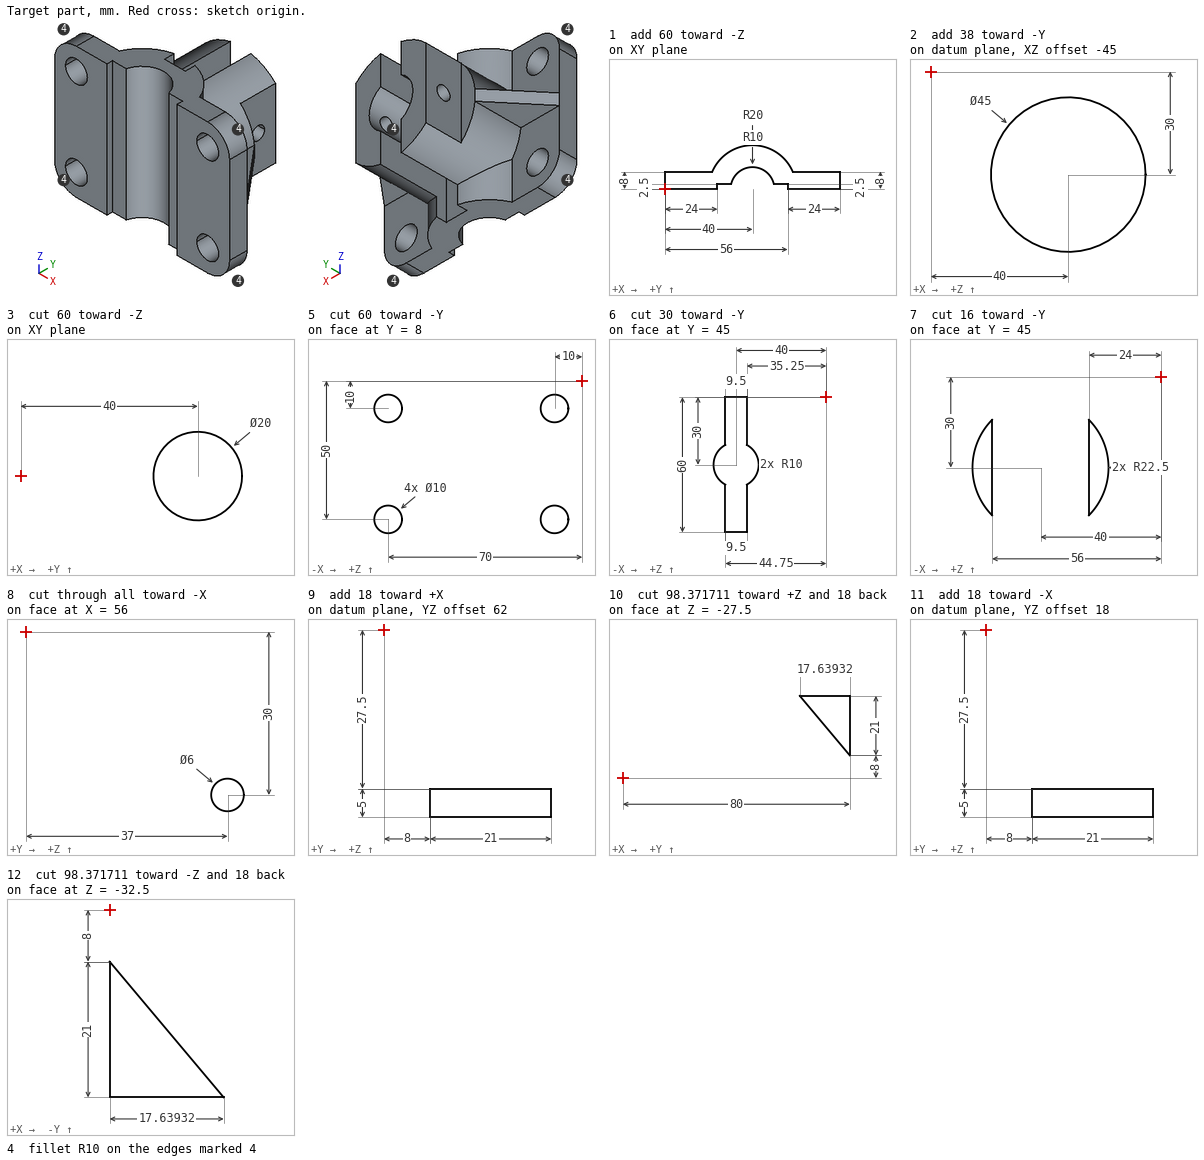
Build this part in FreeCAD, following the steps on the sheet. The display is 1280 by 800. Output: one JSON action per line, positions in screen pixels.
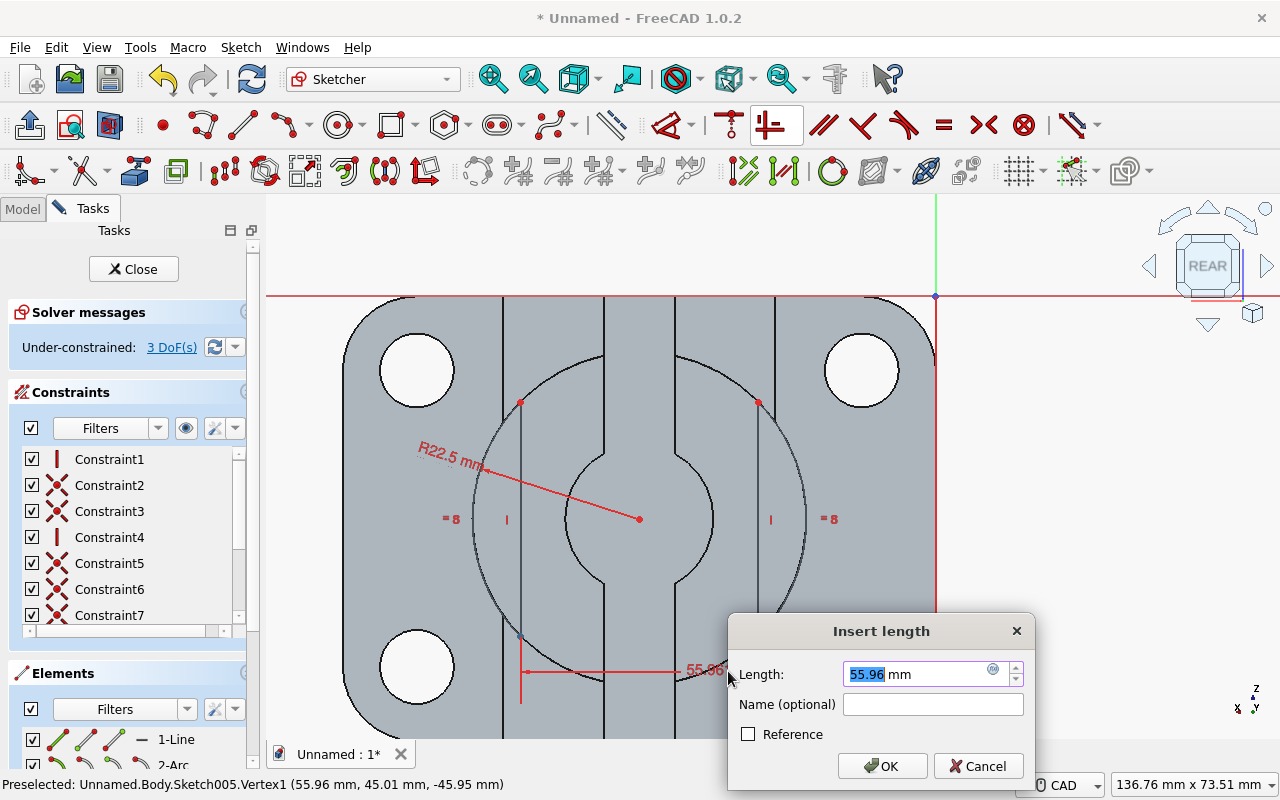
{"action": "type", "text": "56"}
{"action": "key", "text": "Return"}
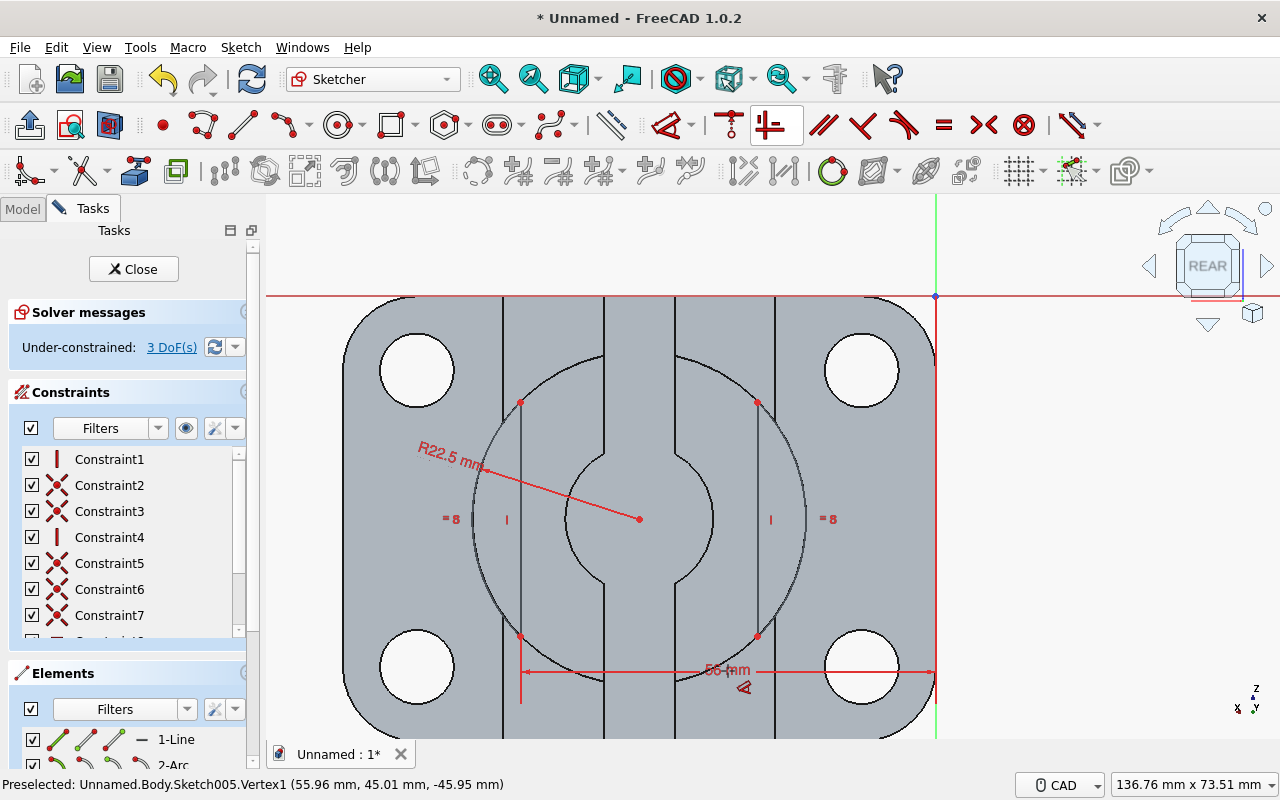
{"action": "left_click", "coordinate": [758, 402]}
{"action": "left_click", "coordinate": [847, 262]}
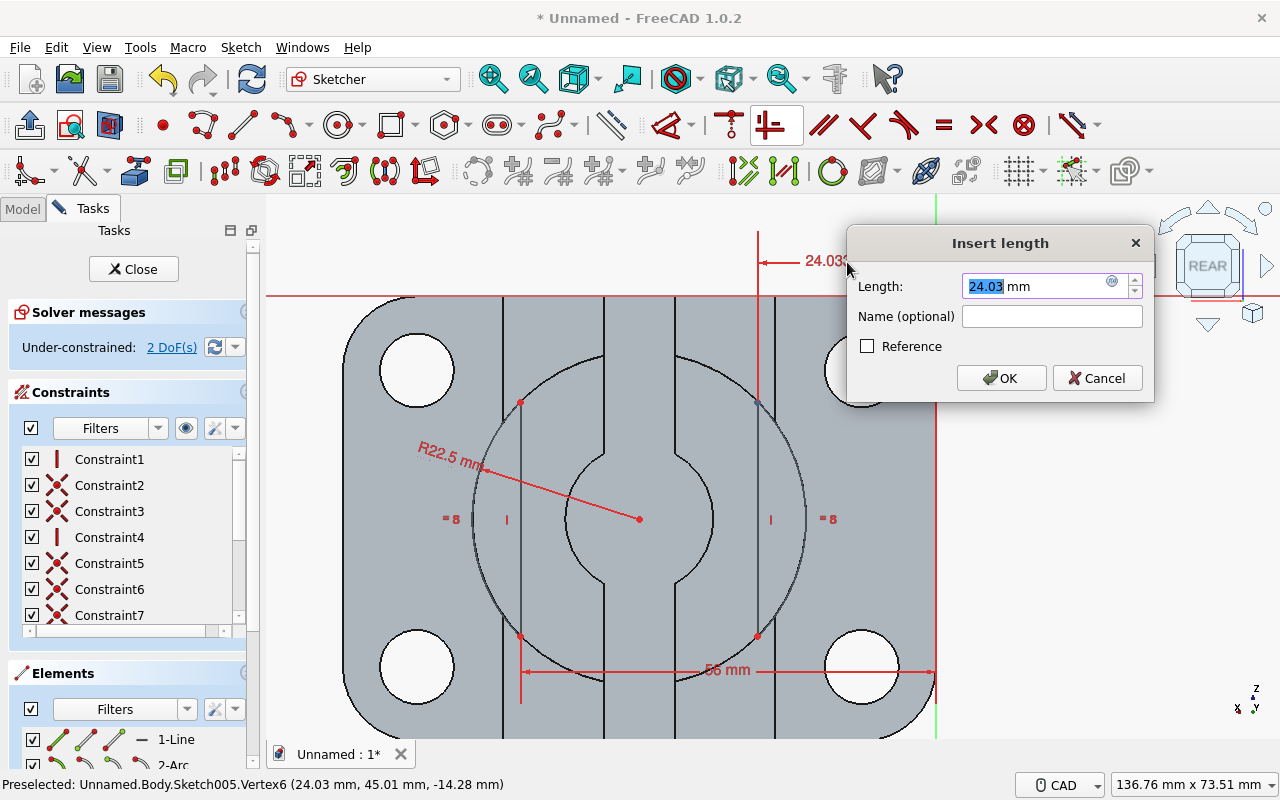
{"action": "type", "text": "24"}
{"action": "key", "text": "Return"}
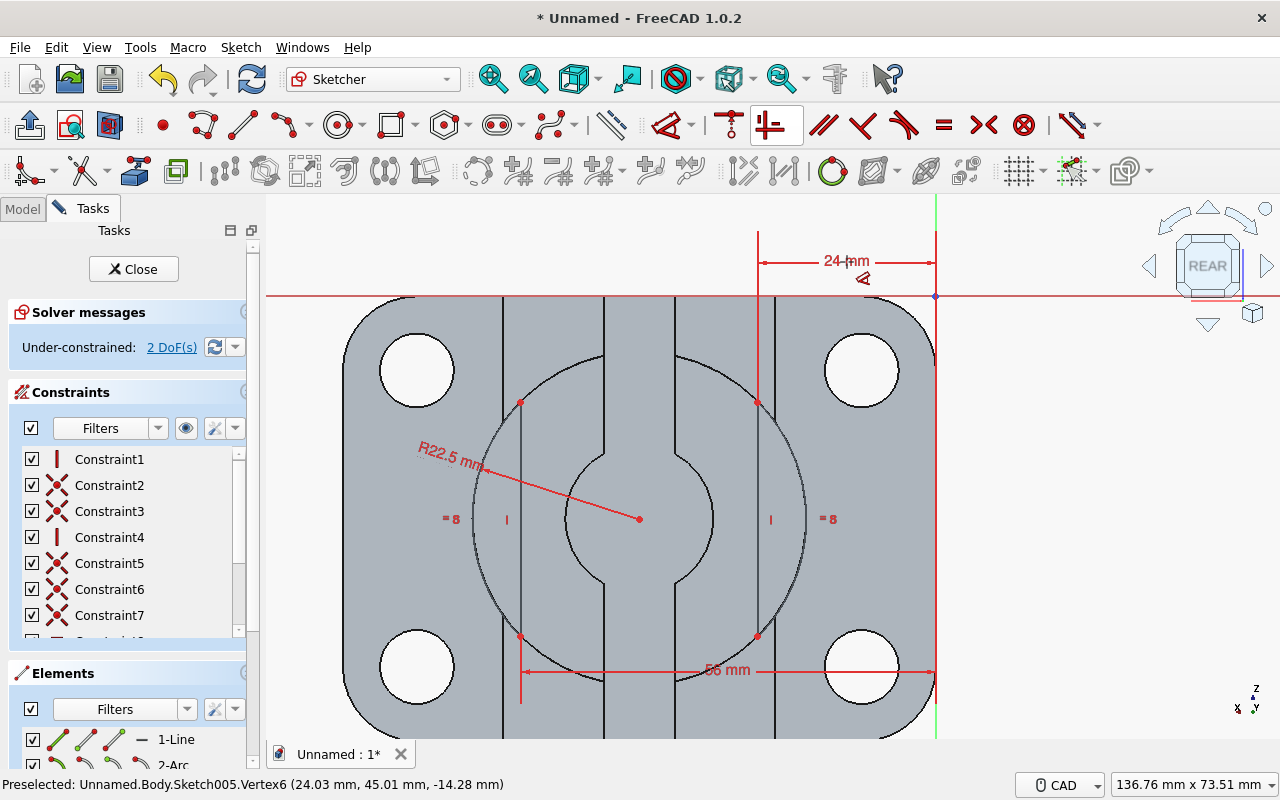
{"action": "left_click", "coordinate": [639, 520]}
{"action": "left_click", "coordinate": [719, 262]}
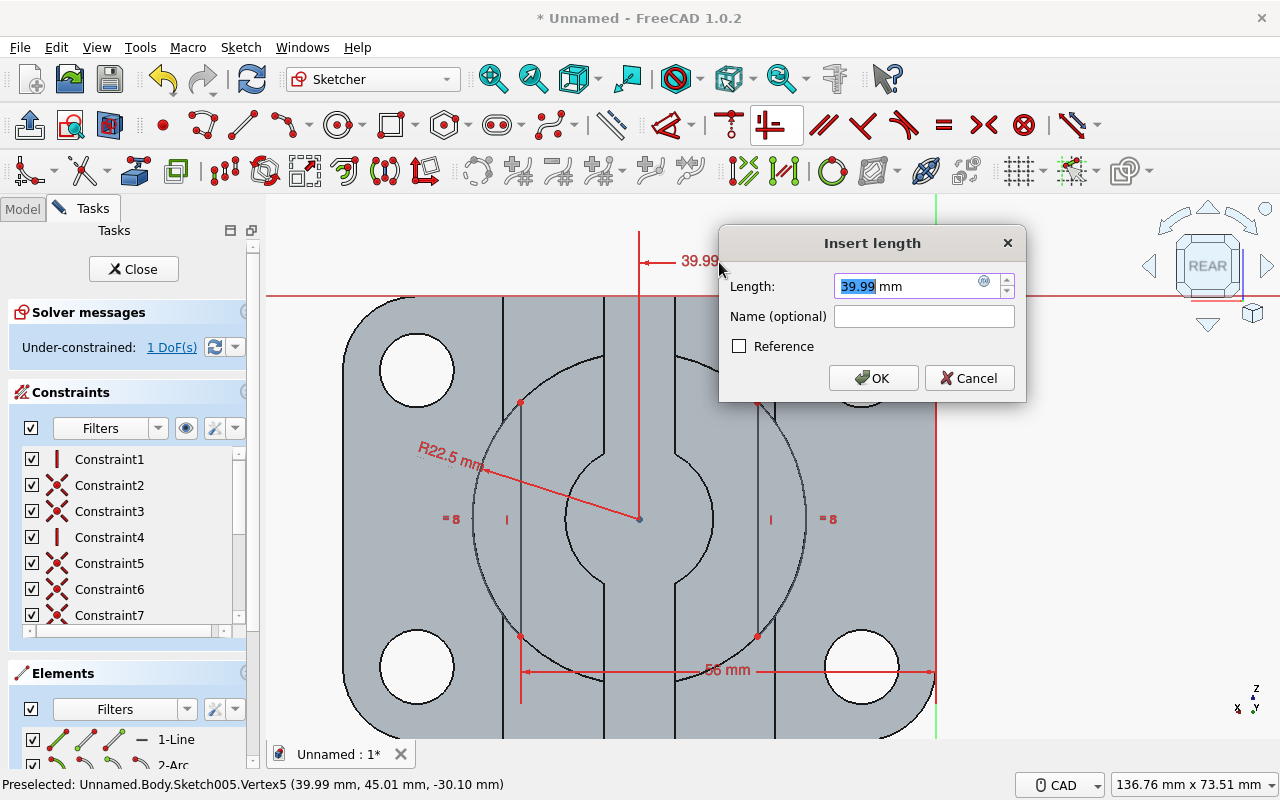
{"action": "type", "text": "40"}
{"action": "key", "text": "Return"}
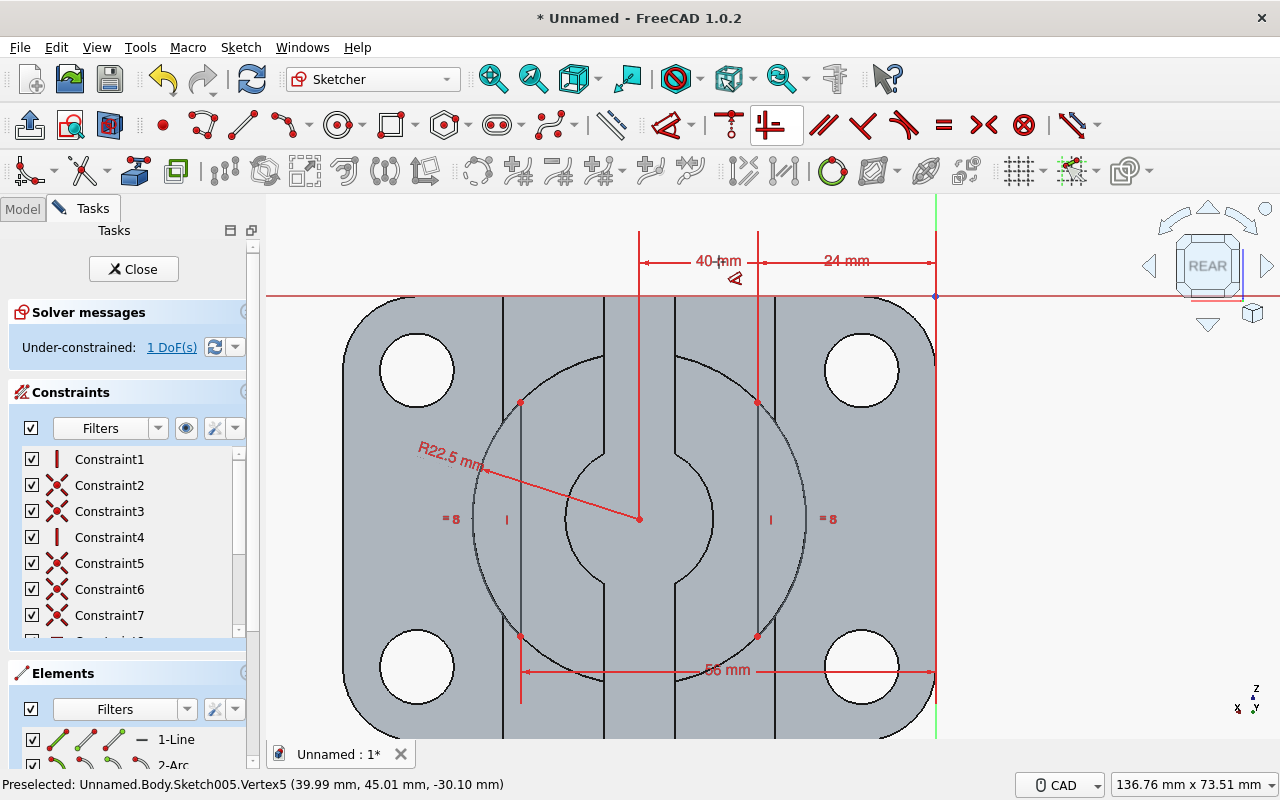
{"action": "left_click", "coordinate": [639, 520]}
{"action": "left_click", "coordinate": [970, 408]}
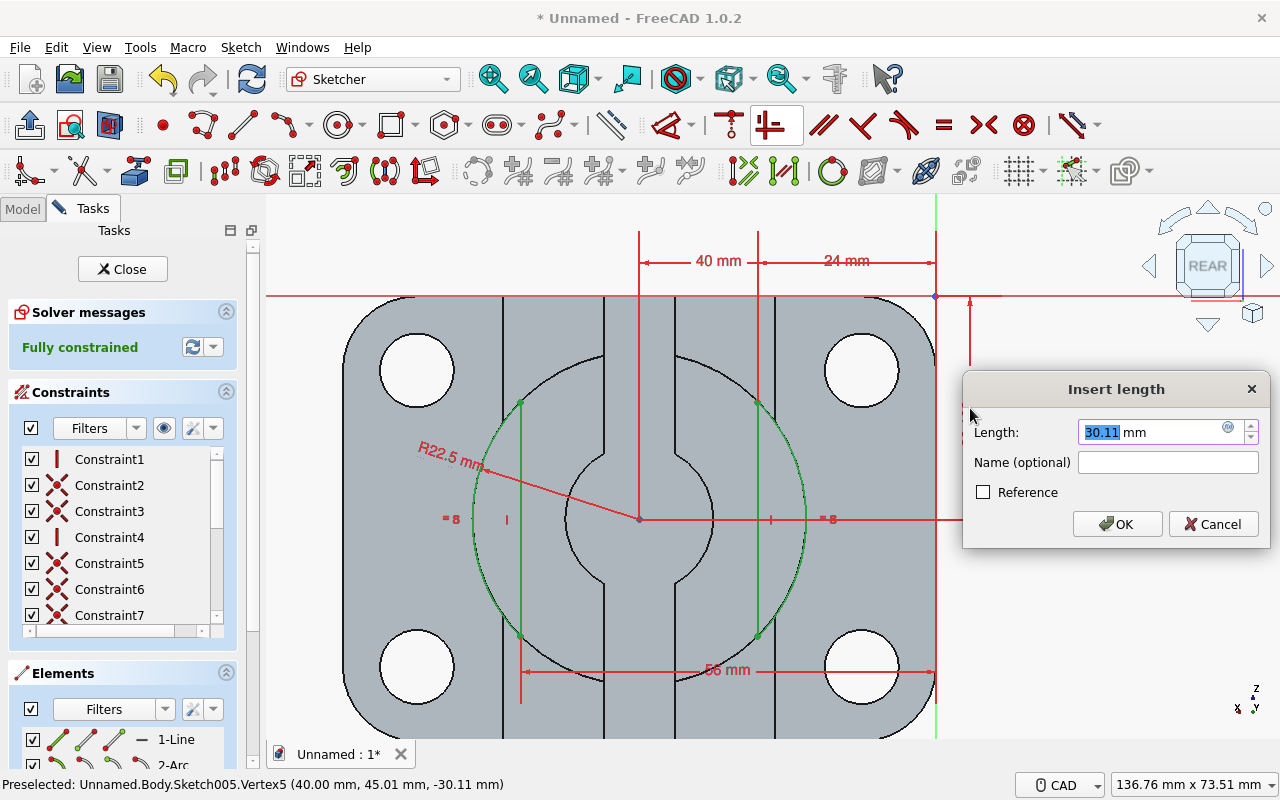
{"action": "type", "text": "30"}
{"action": "key", "text": "Return"}
{"action": "key", "text": "Escape"}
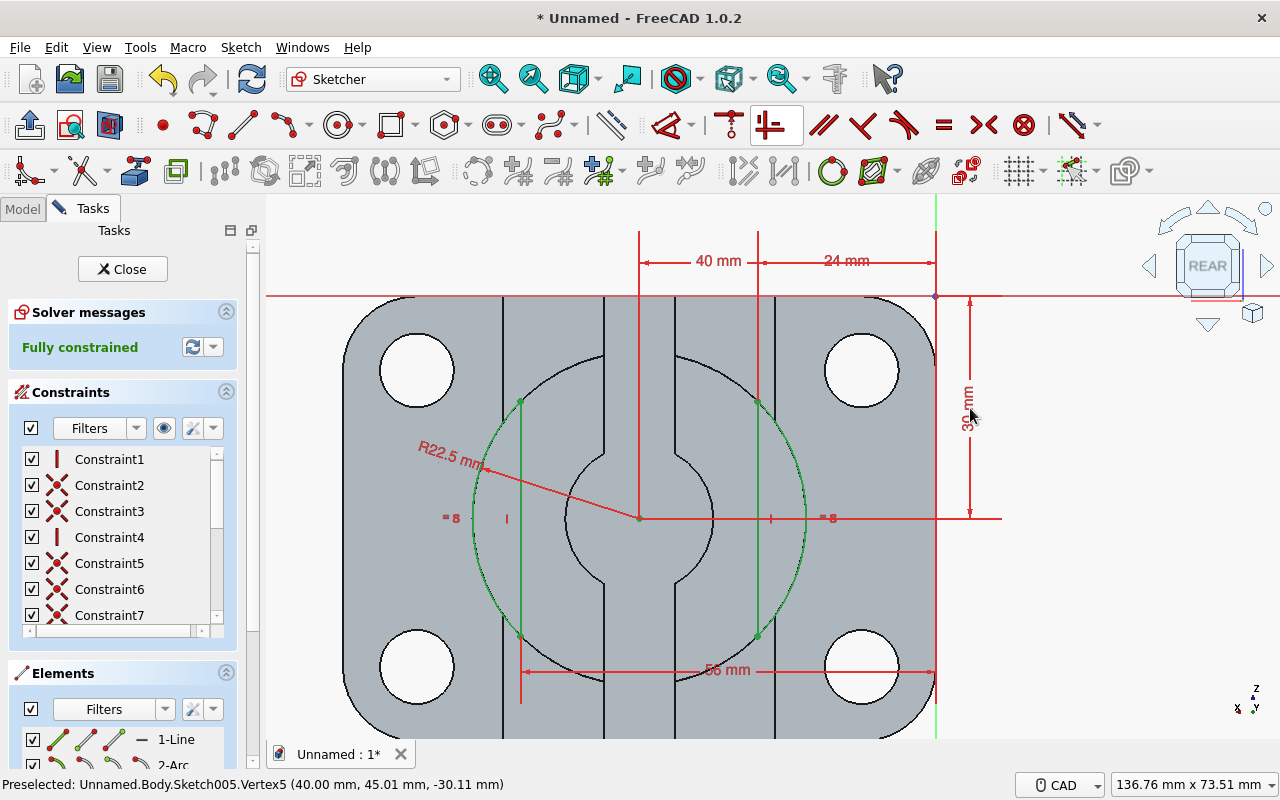
{"action": "left_click", "coordinate": [123, 269]}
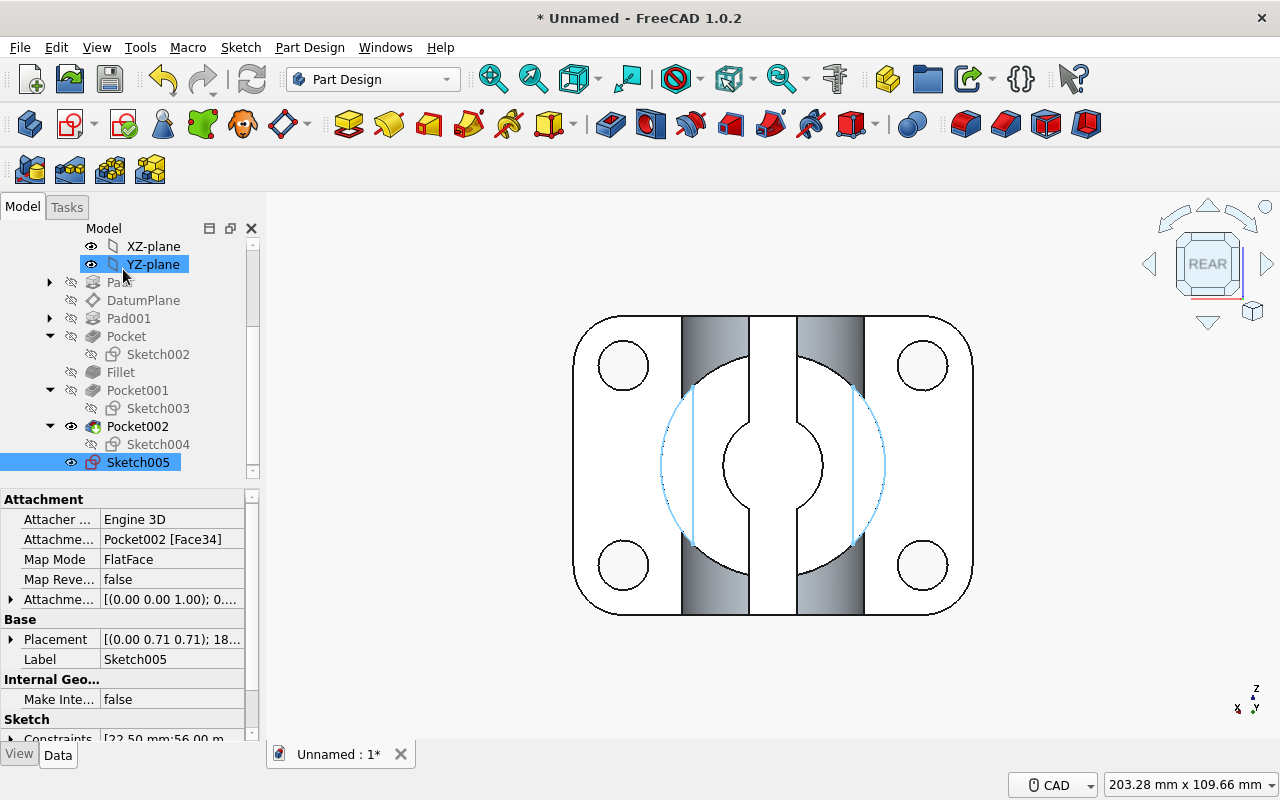
{"action": "left_click", "coordinate": [612, 124]}